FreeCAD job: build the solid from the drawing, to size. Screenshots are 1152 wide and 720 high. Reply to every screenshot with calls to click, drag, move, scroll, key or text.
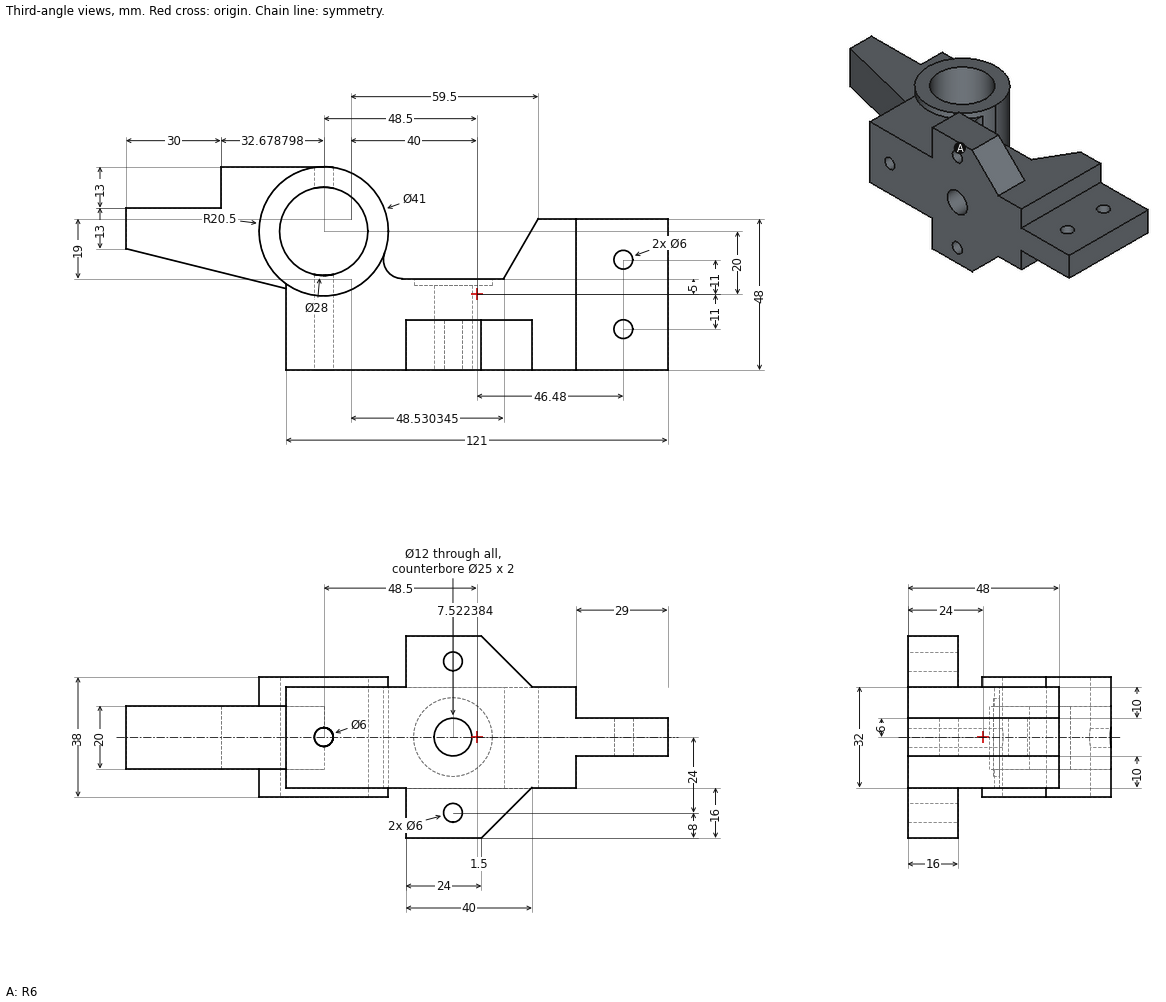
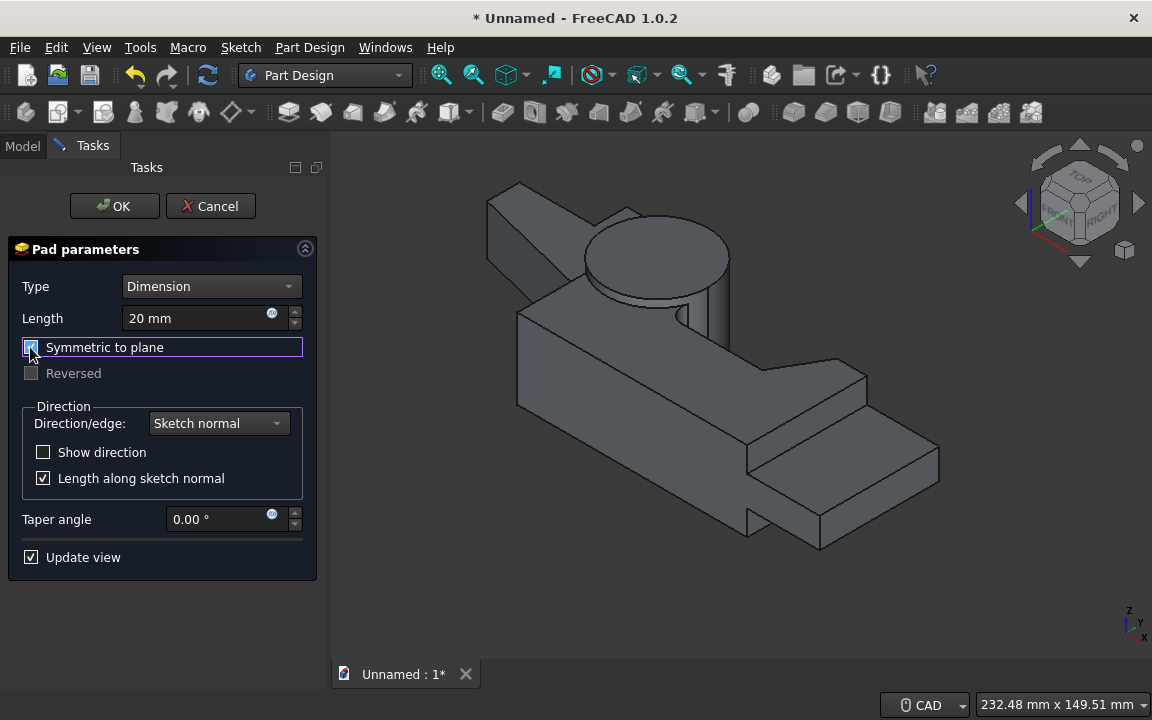
click(115, 206)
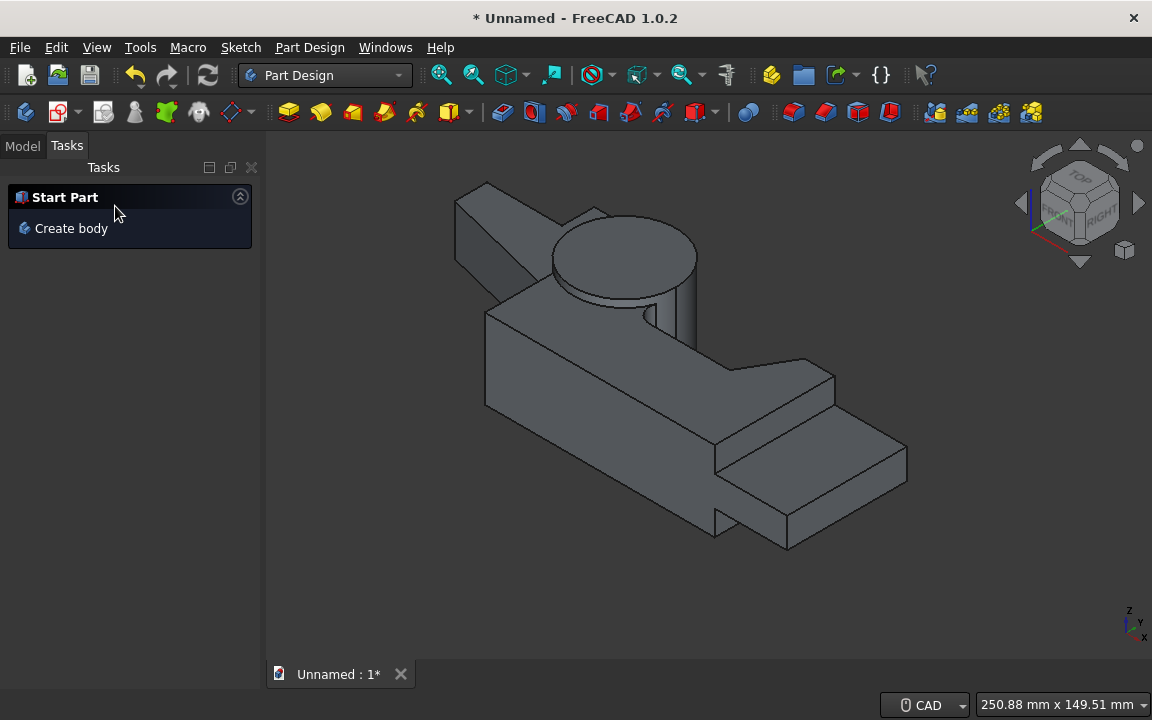
click(58, 112)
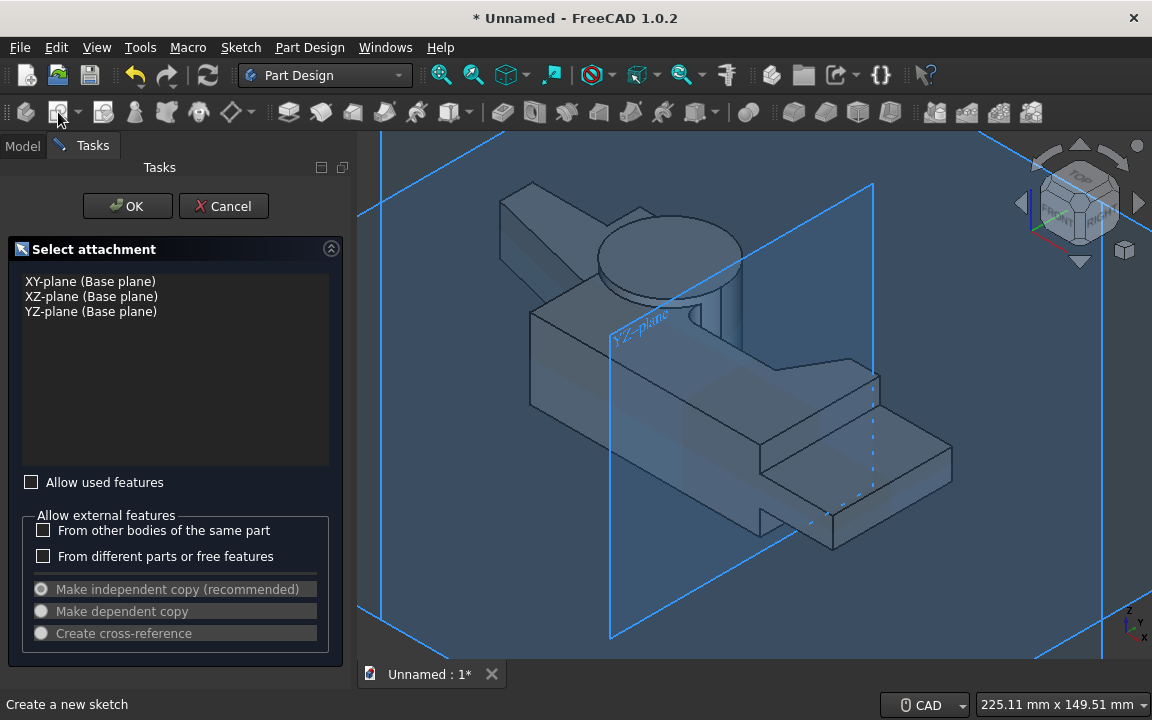
click(82, 296)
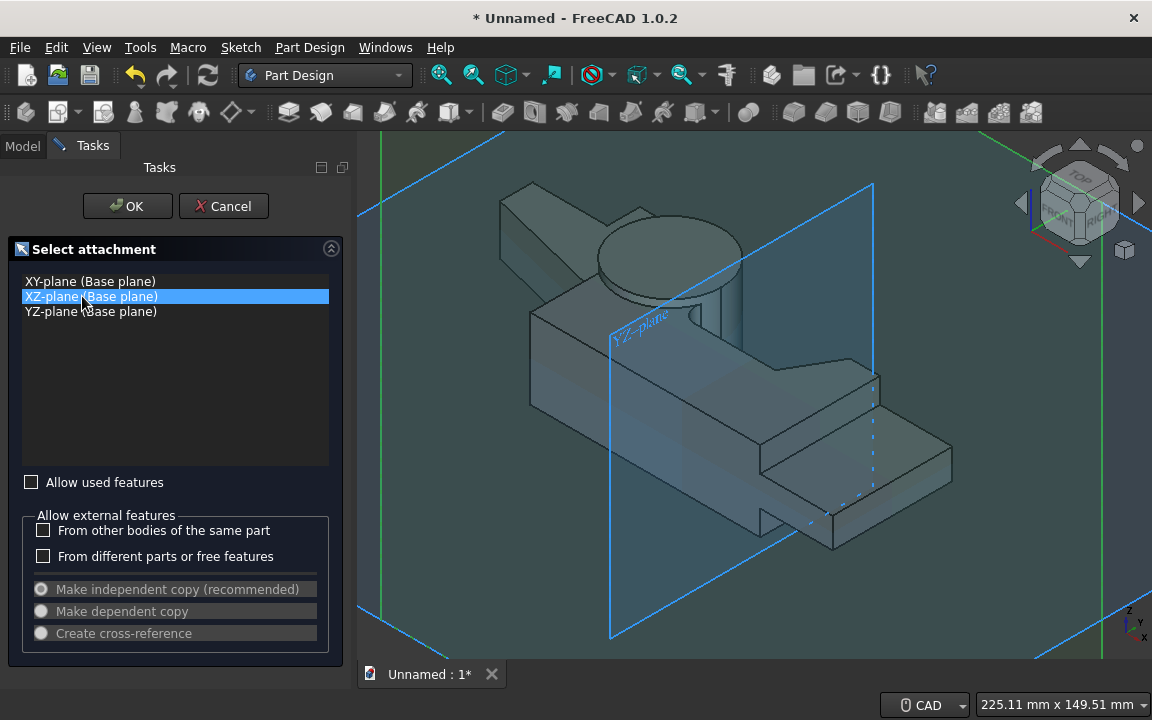
click(128, 206)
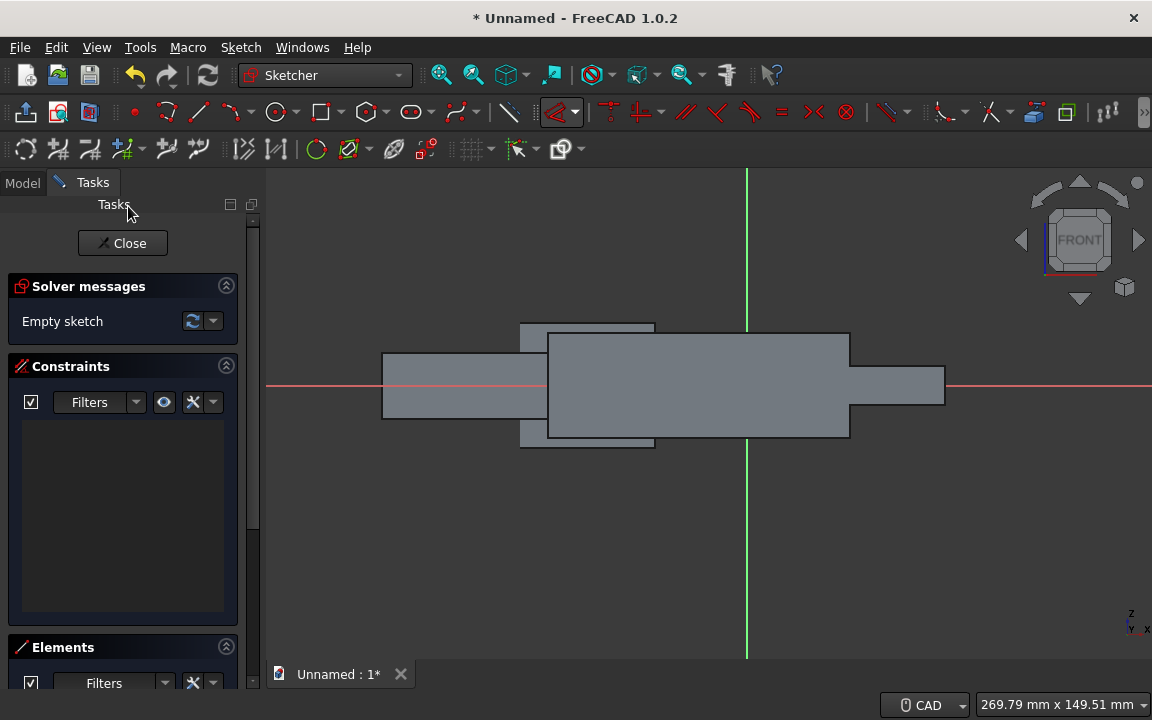
key(q)
key(s)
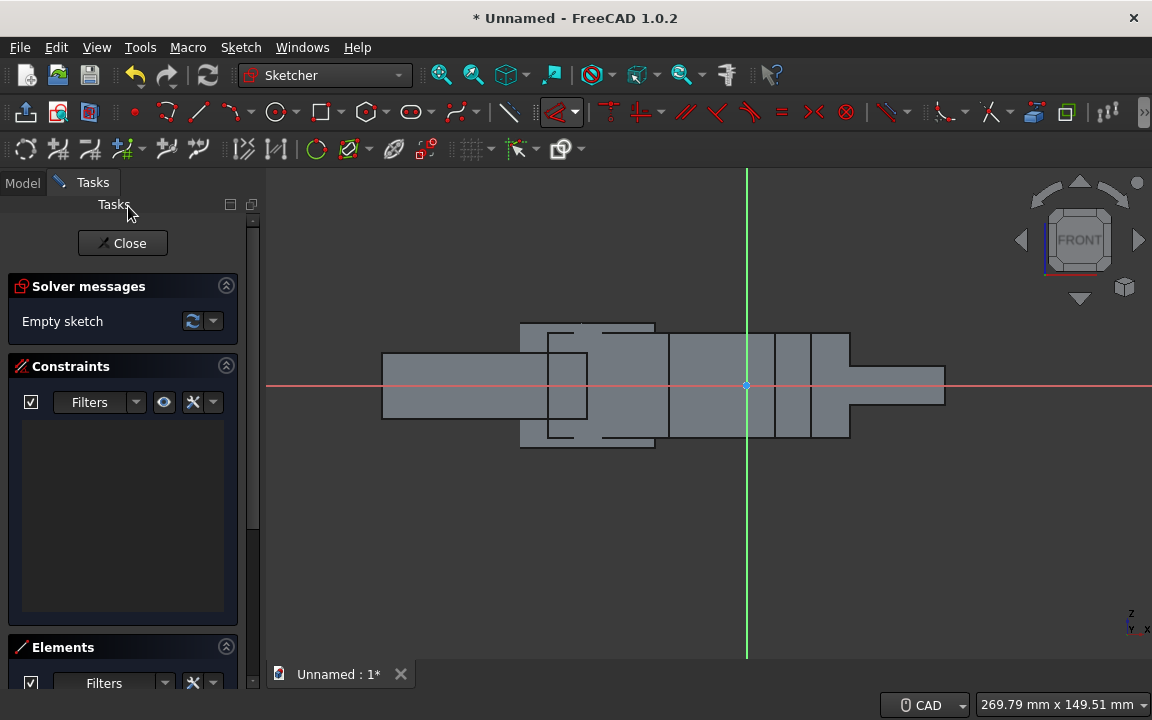
scroll(584, 384, up, 14)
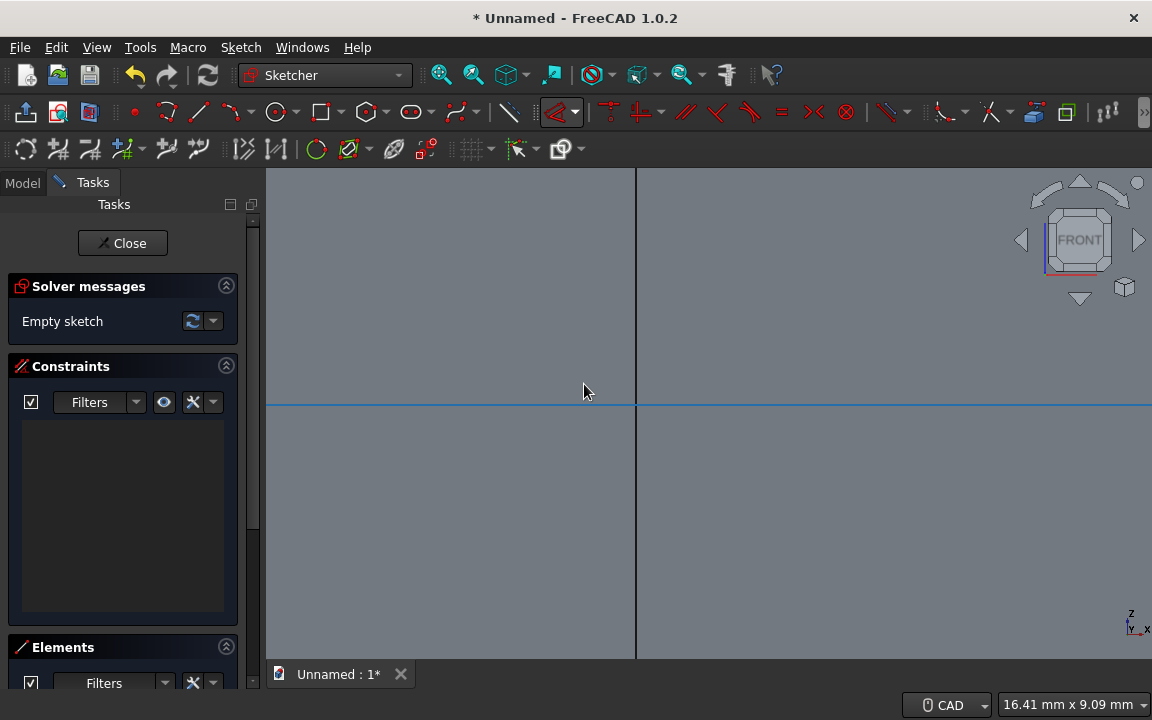
key(g)
key(c)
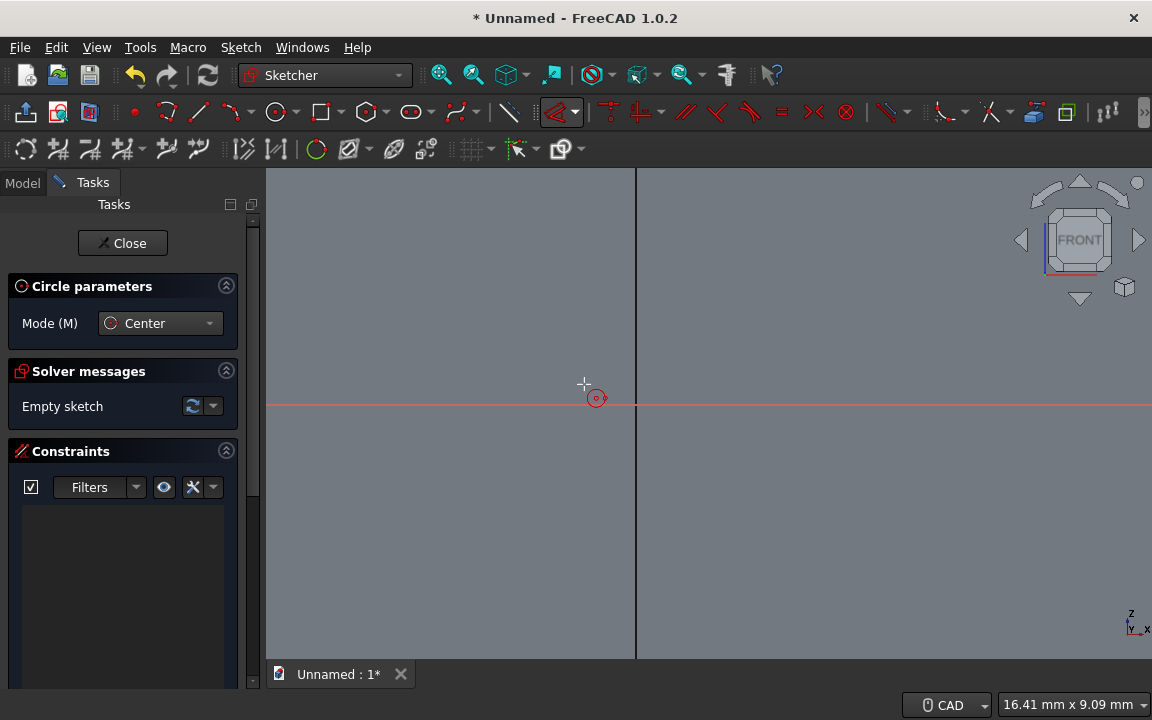
click(636, 405)
move(750, 290)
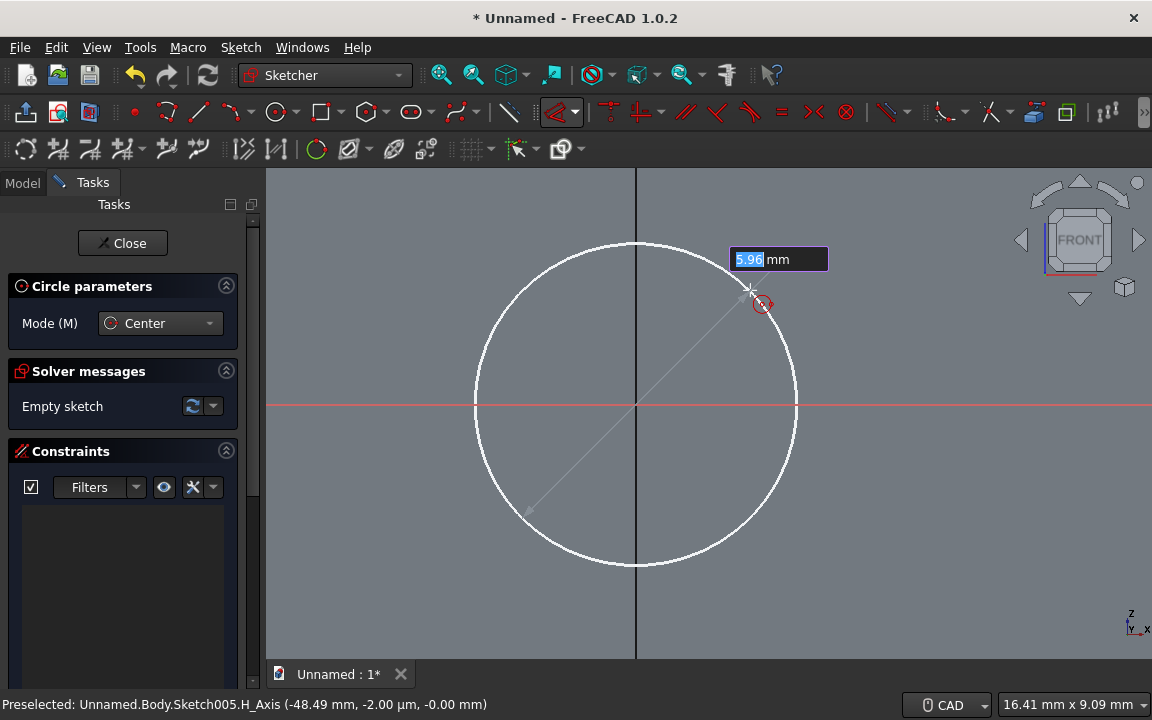
text(6)
key(Return)
key(Escape)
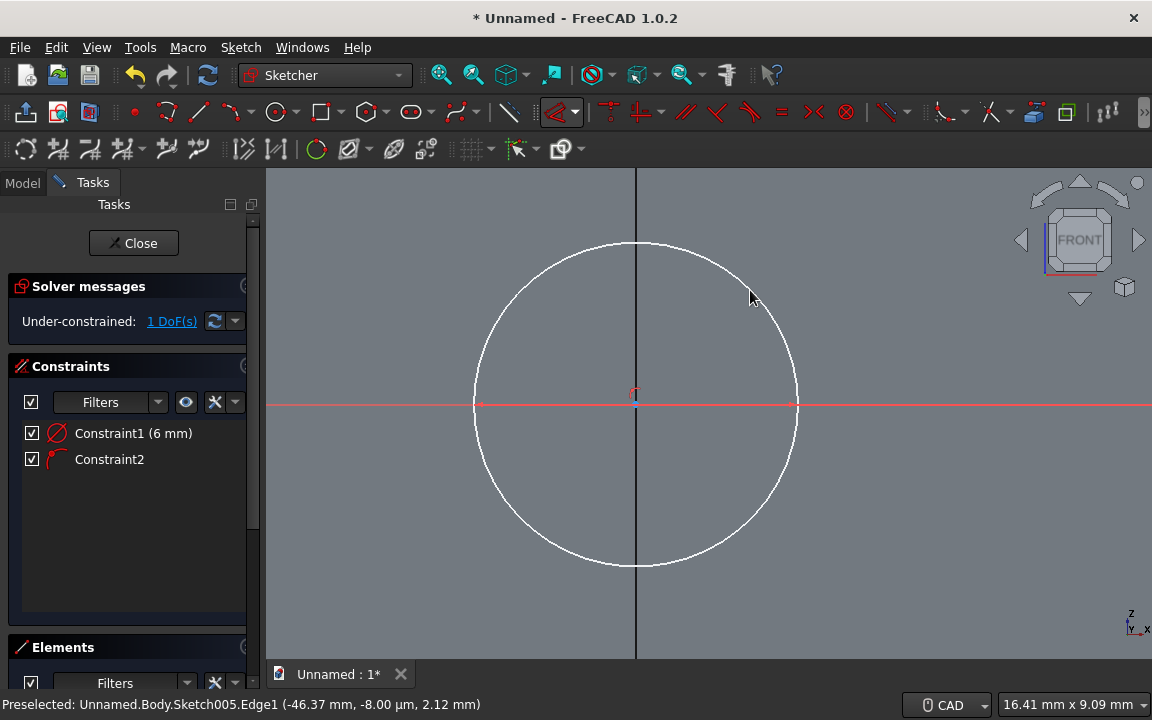
click(636, 405)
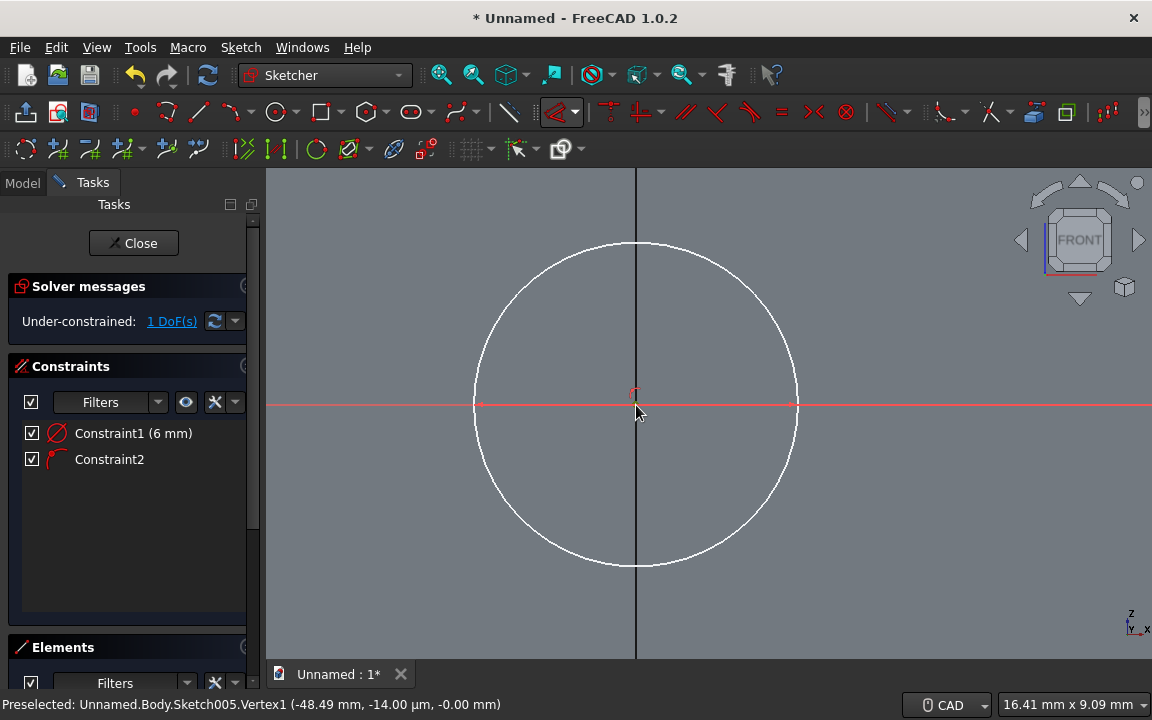
key(l)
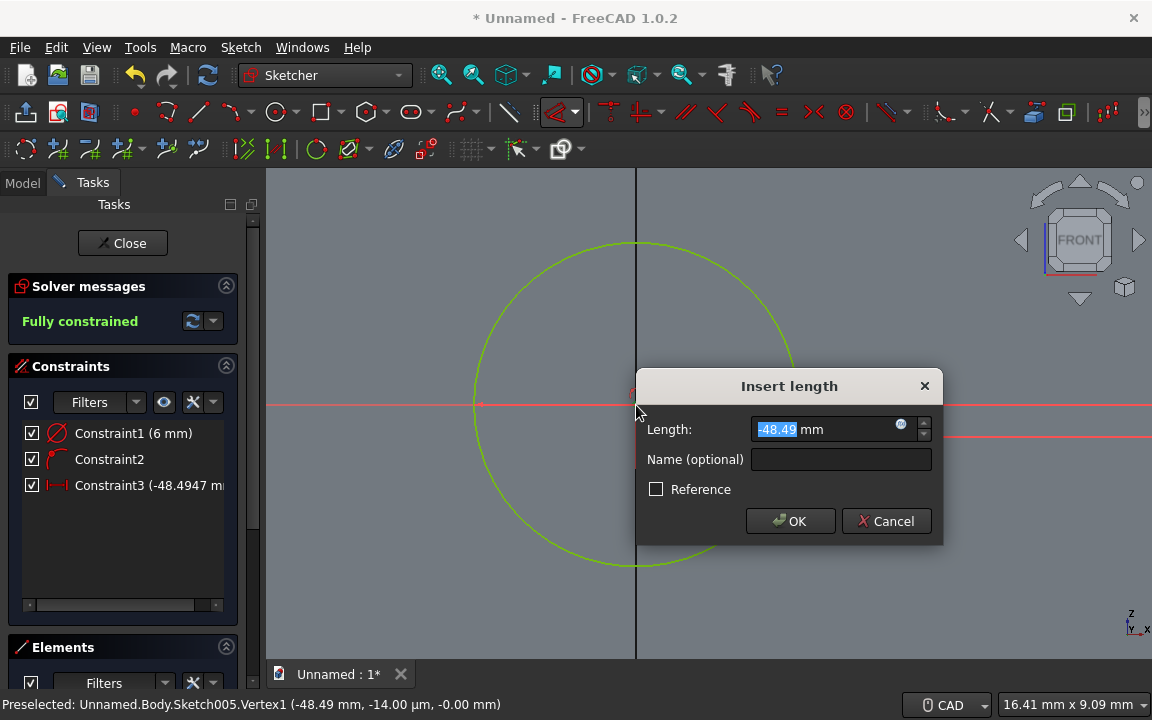
text(-48.5)
key(Return)